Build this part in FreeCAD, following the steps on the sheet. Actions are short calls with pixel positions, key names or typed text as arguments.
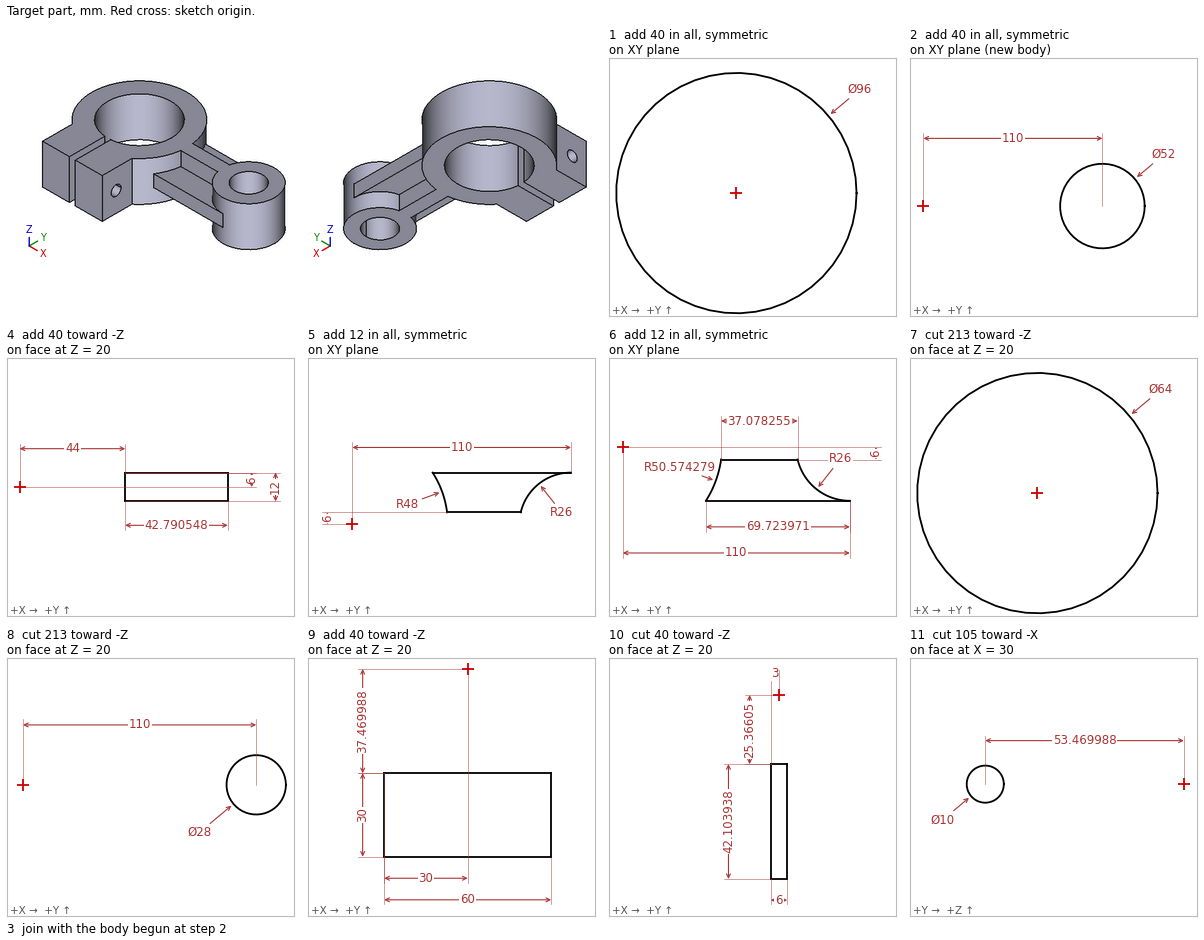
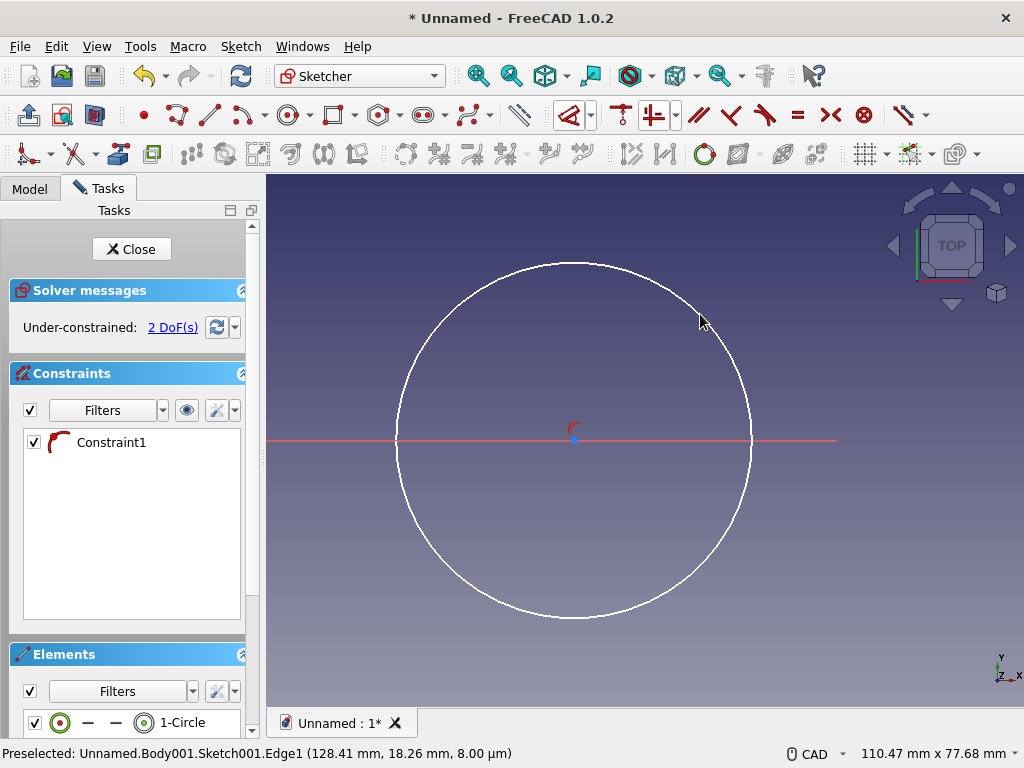
click(699, 314)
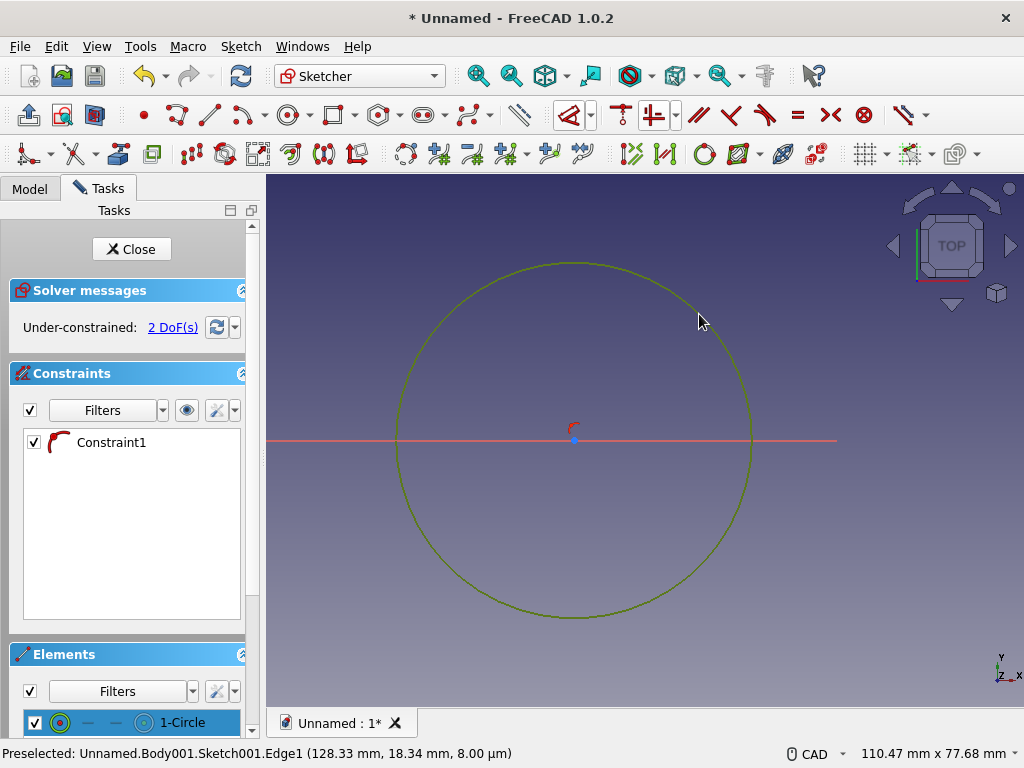
key(k)
key(o)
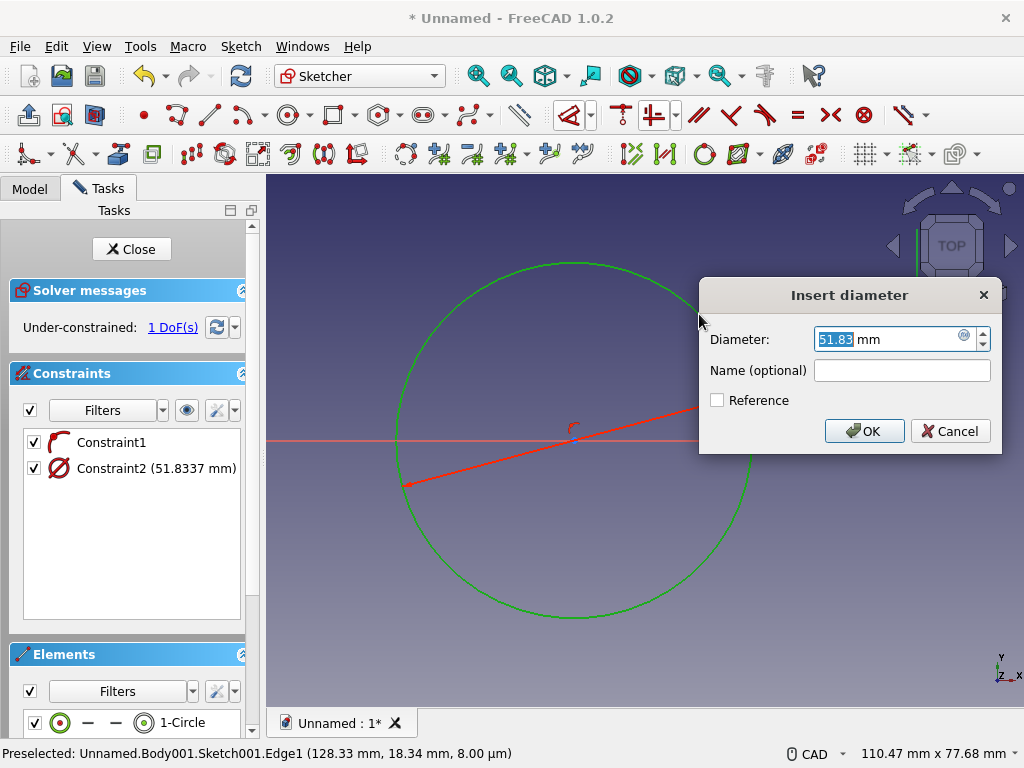
text(52)
key(Return)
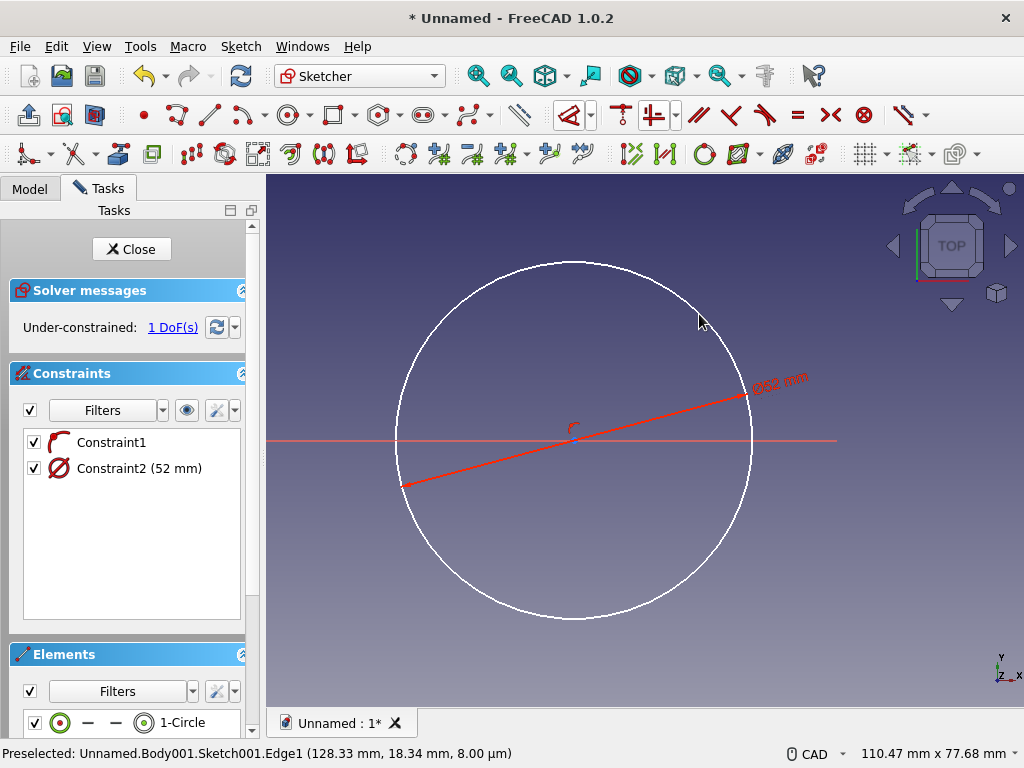
click(574, 440)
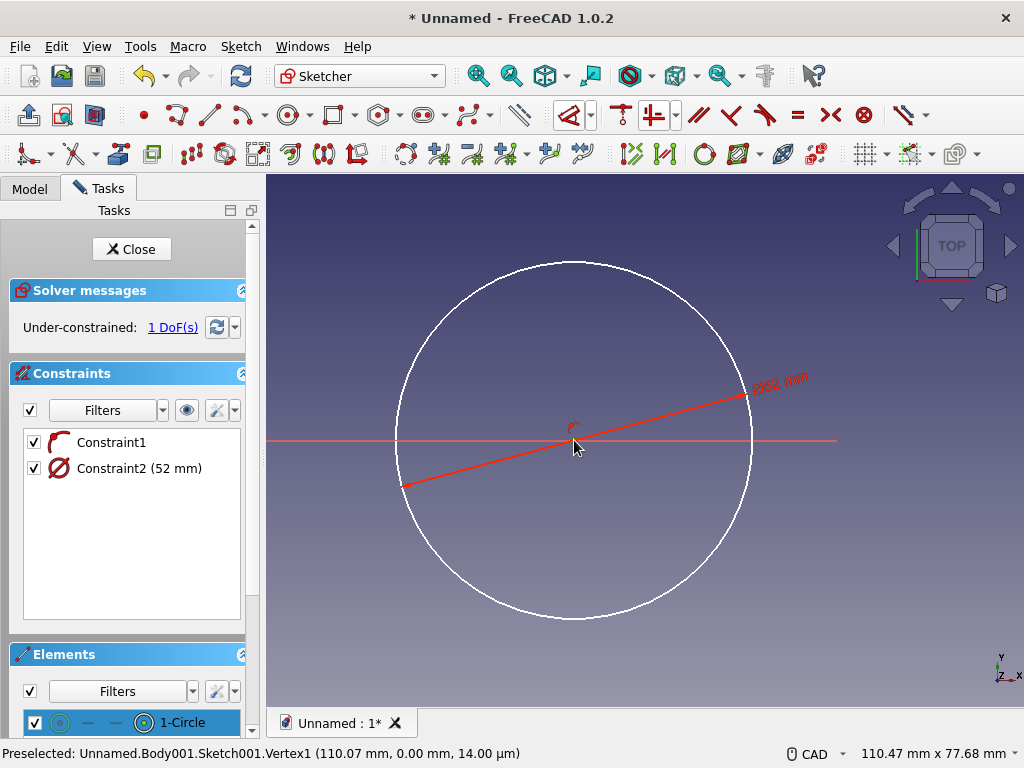
click(590, 116)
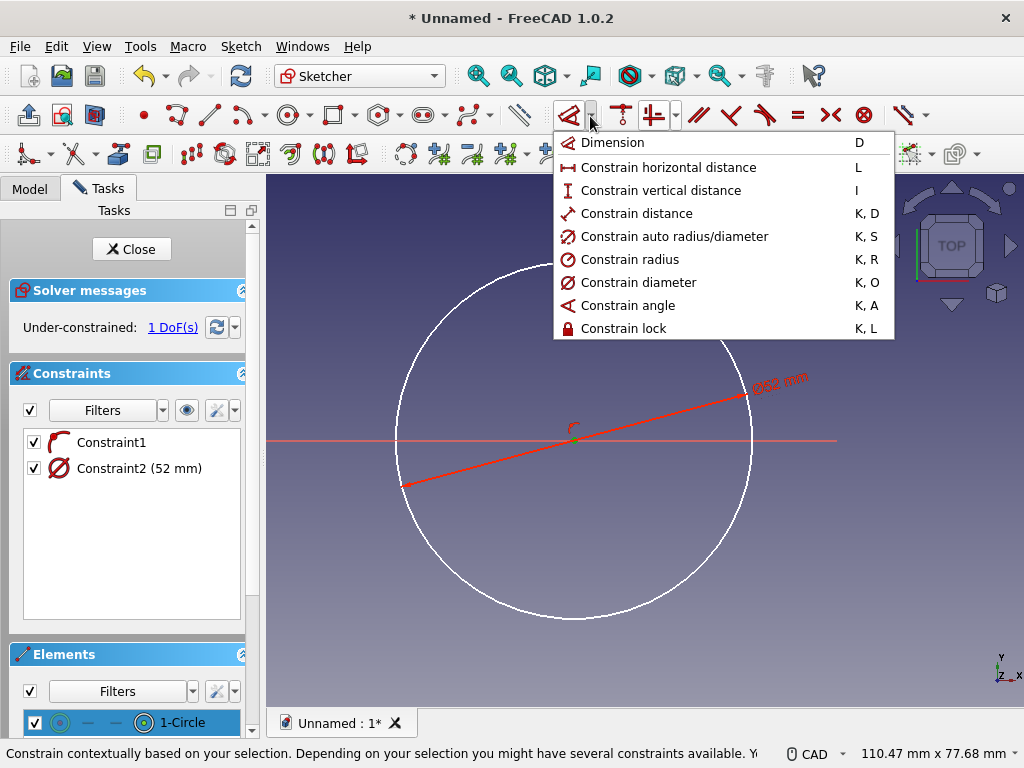
click(724, 168)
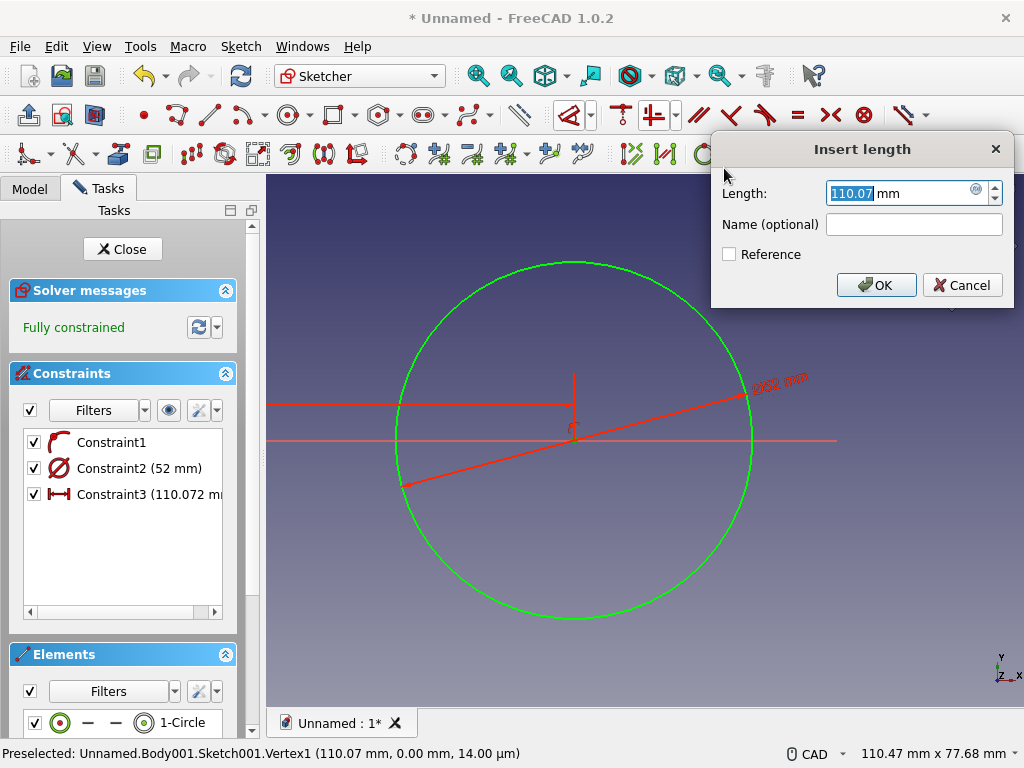
text(110)
key(Return)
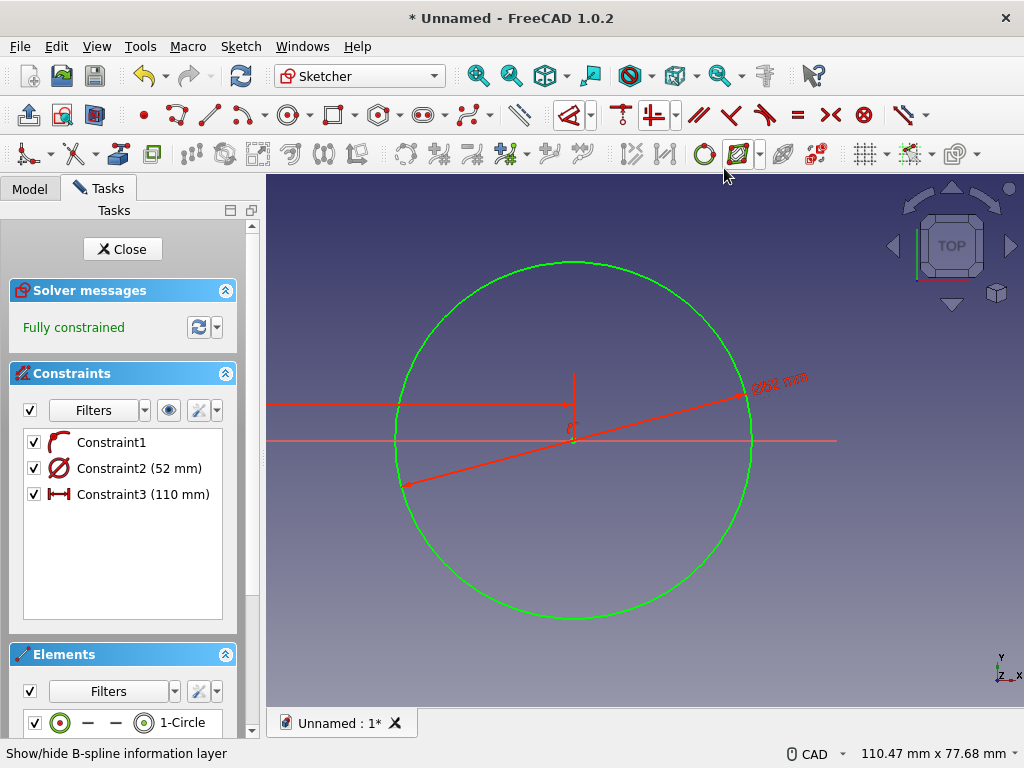
click(123, 249)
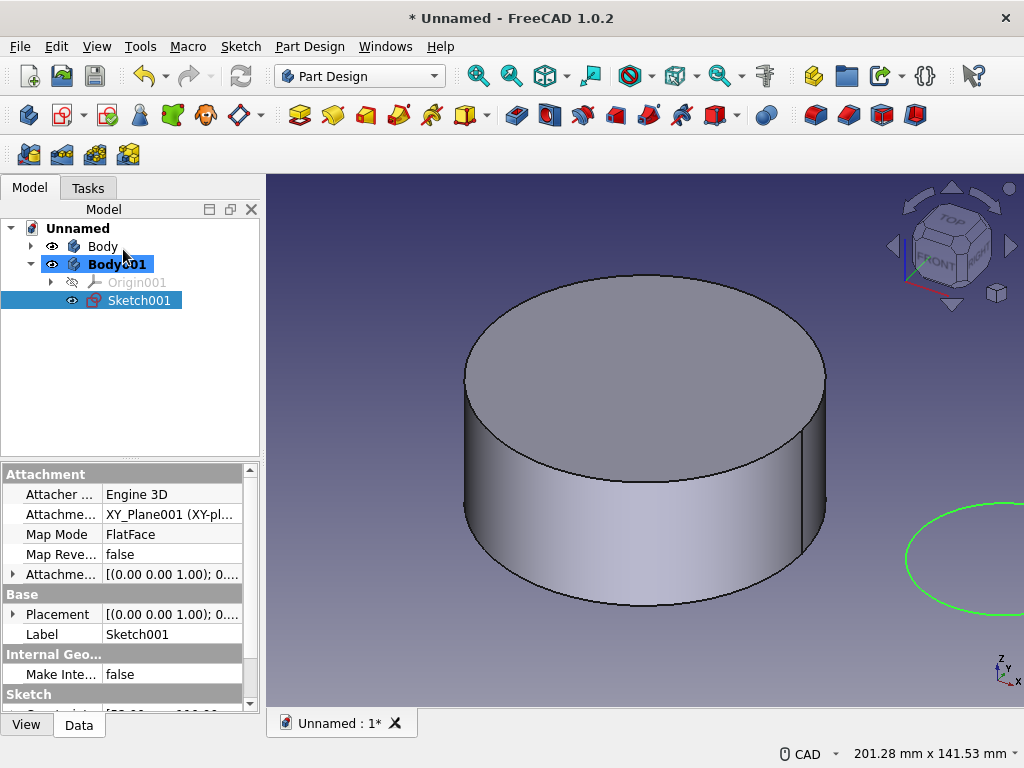
click(300, 116)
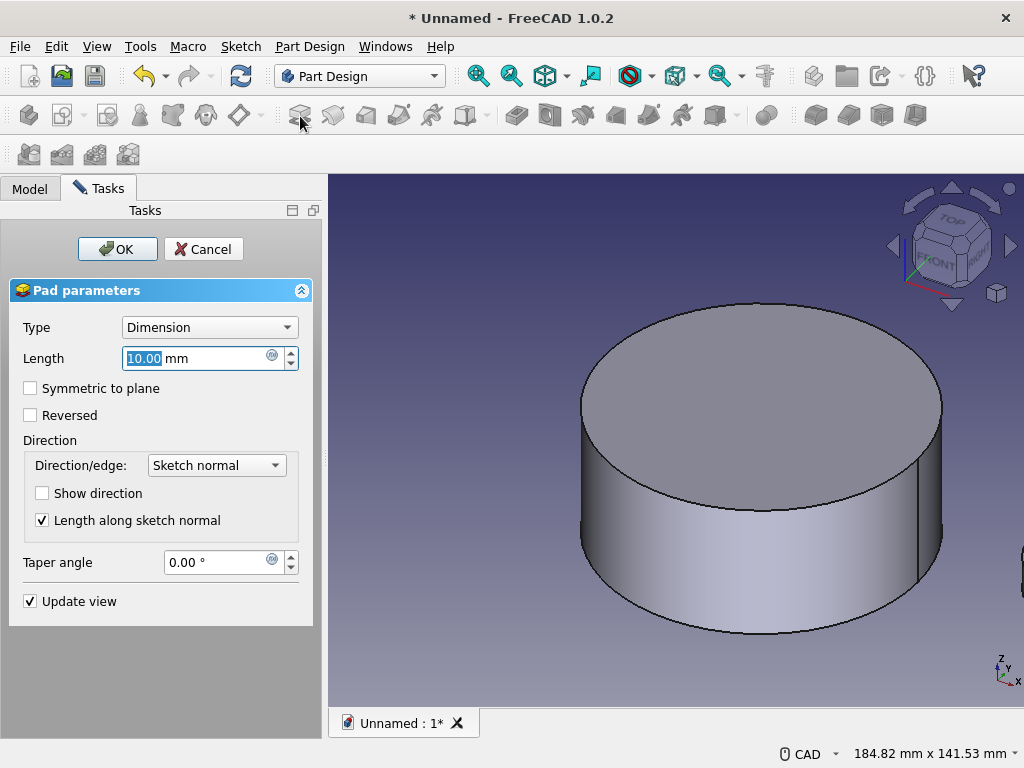
text(40)
key(Tab)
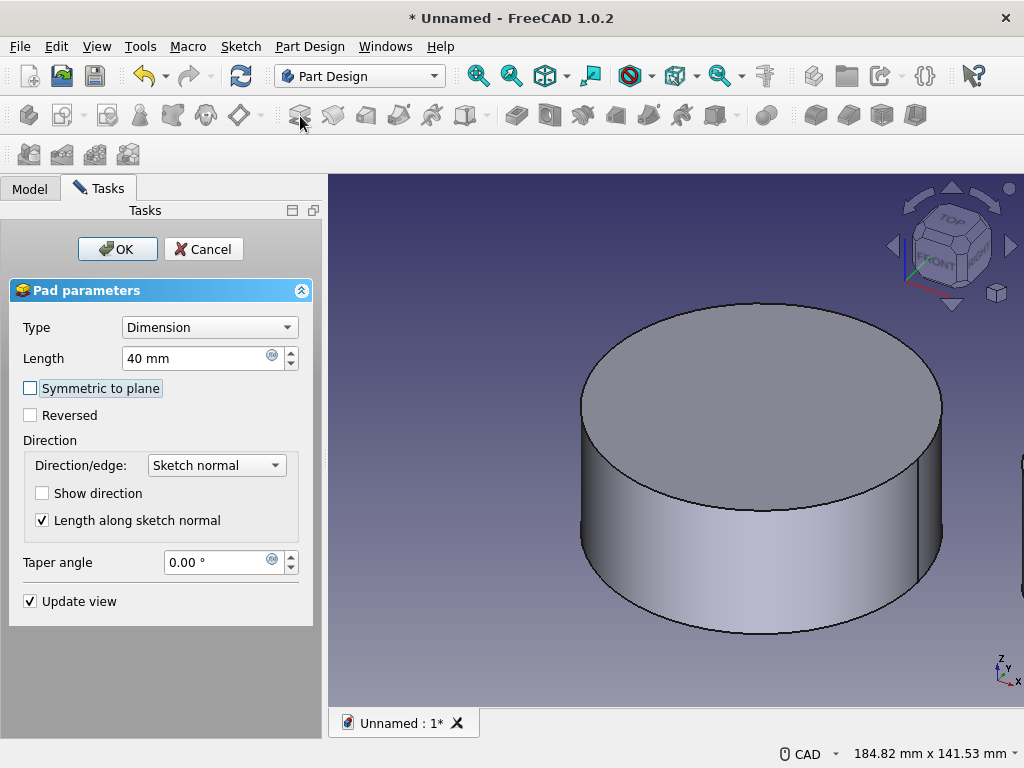
click(31, 388)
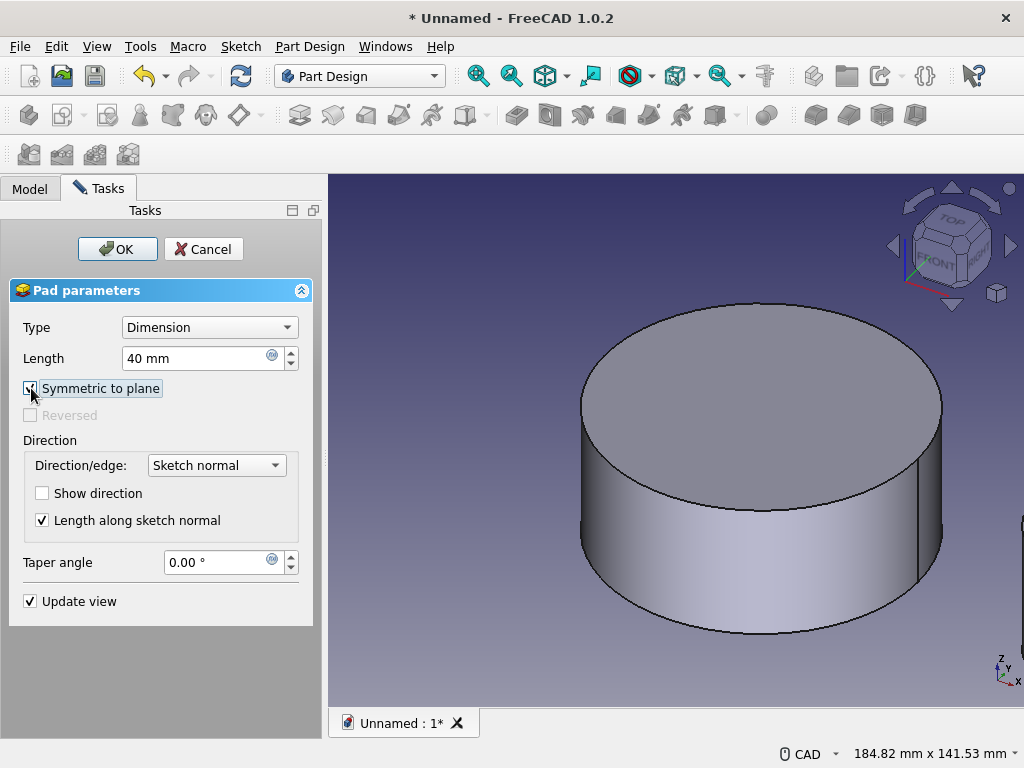
click(118, 249)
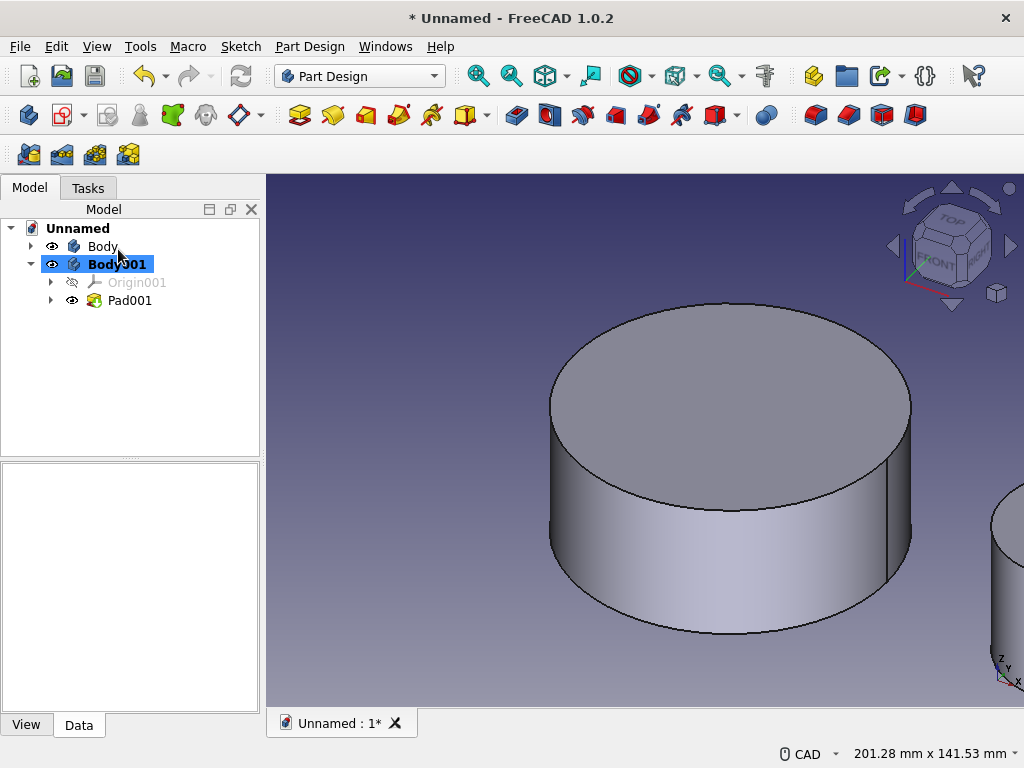
click(479, 76)